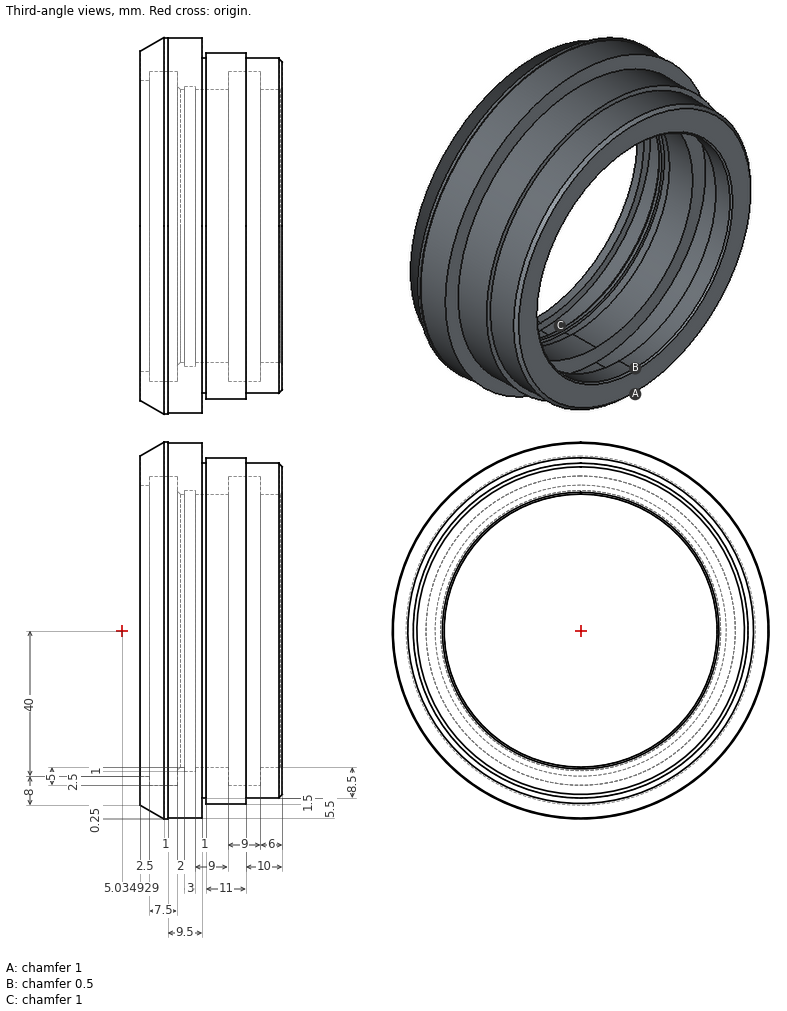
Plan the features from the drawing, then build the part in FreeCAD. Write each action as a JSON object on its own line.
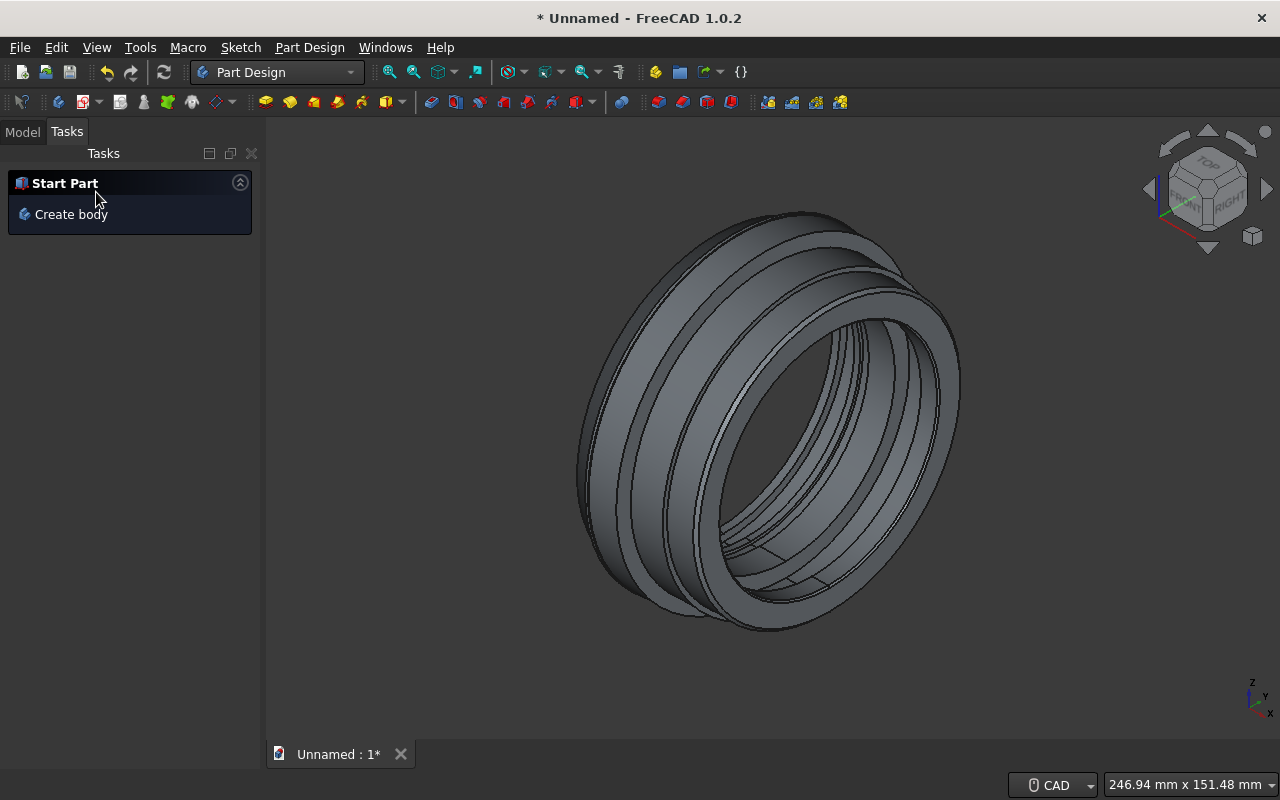
{"action": "key", "text": "2"}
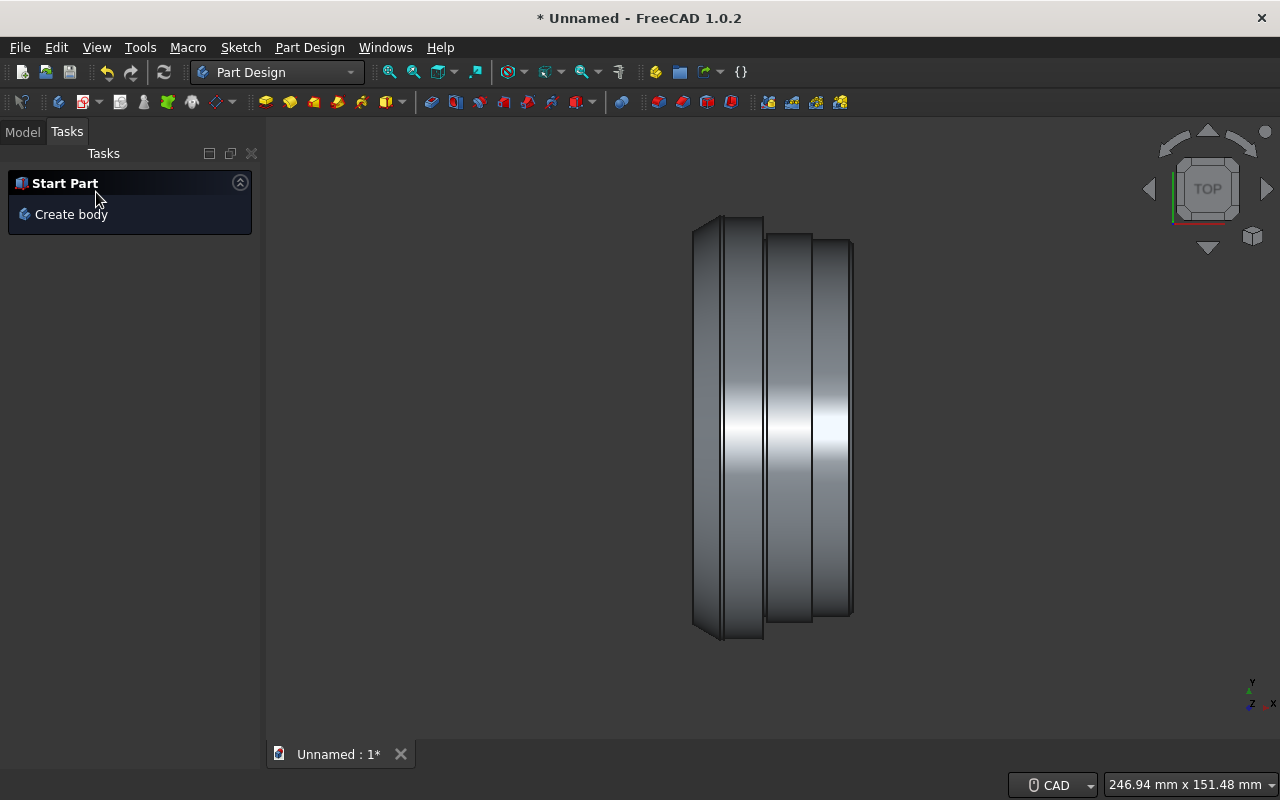
{"action": "key", "text": "1"}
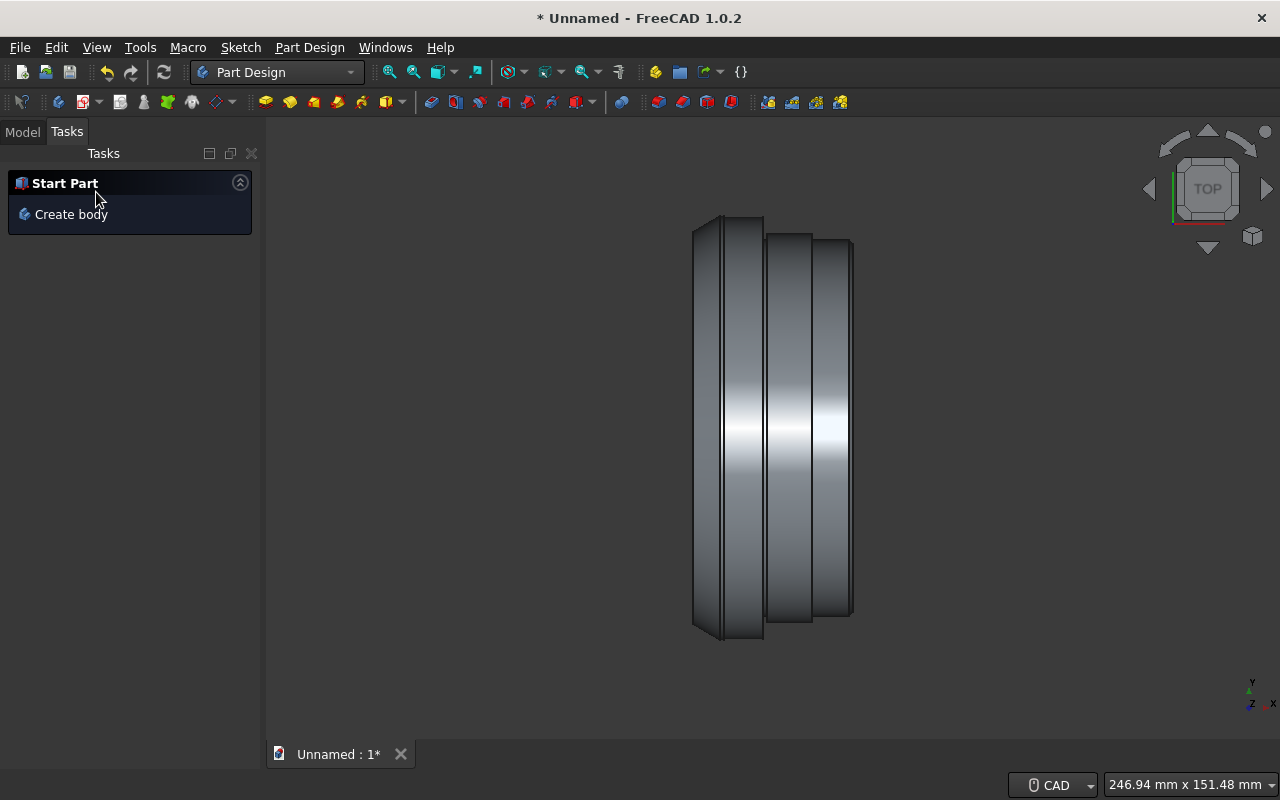
{"action": "key", "text": "3"}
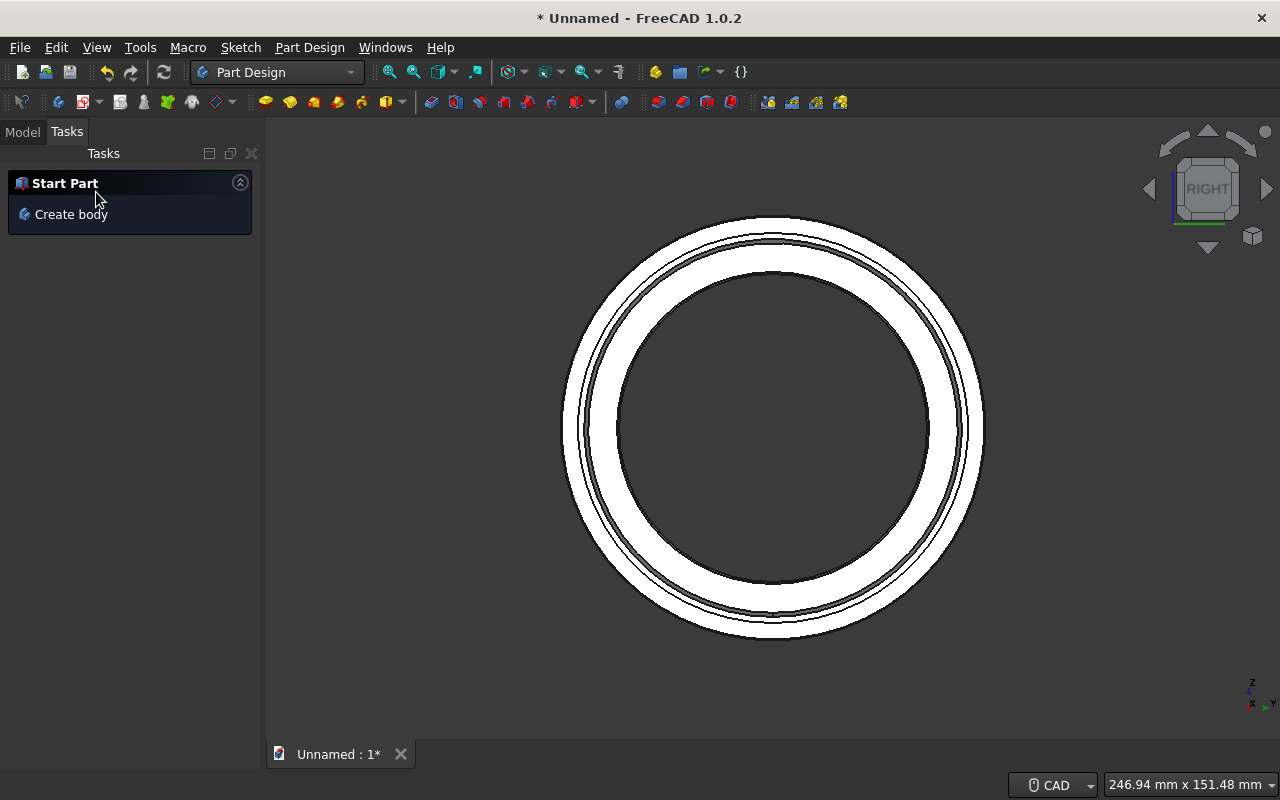
{"action": "key", "text": "5"}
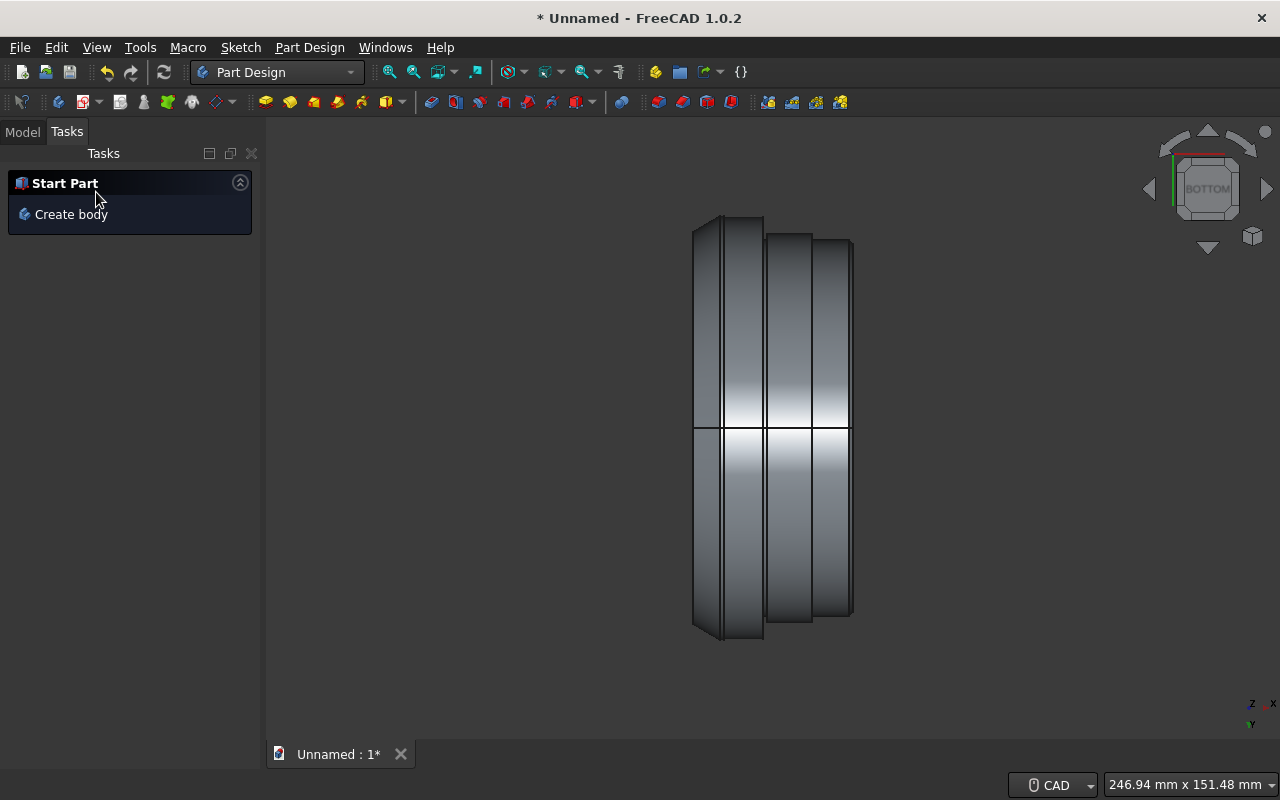
{"action": "key", "text": "4"}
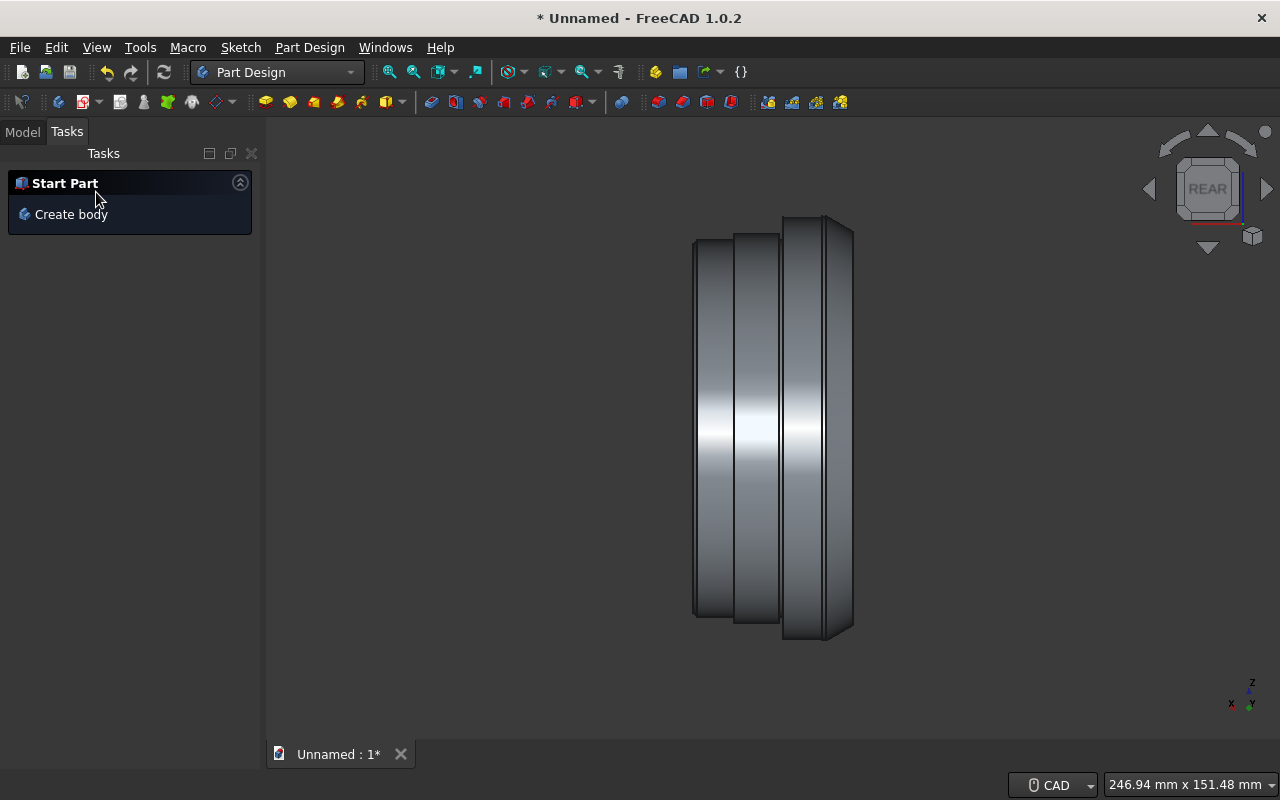
{"action": "key", "text": "6"}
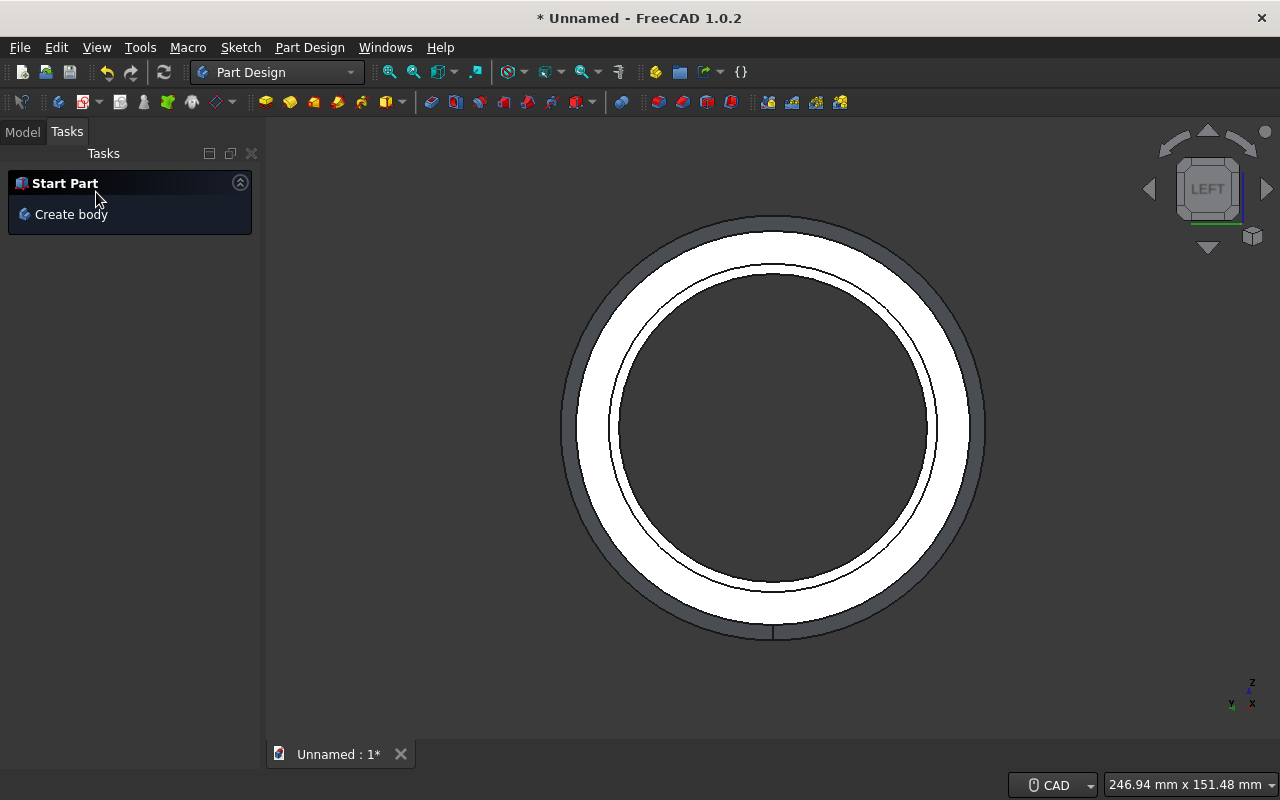
{"action": "left_click", "coordinate": [773, 273]}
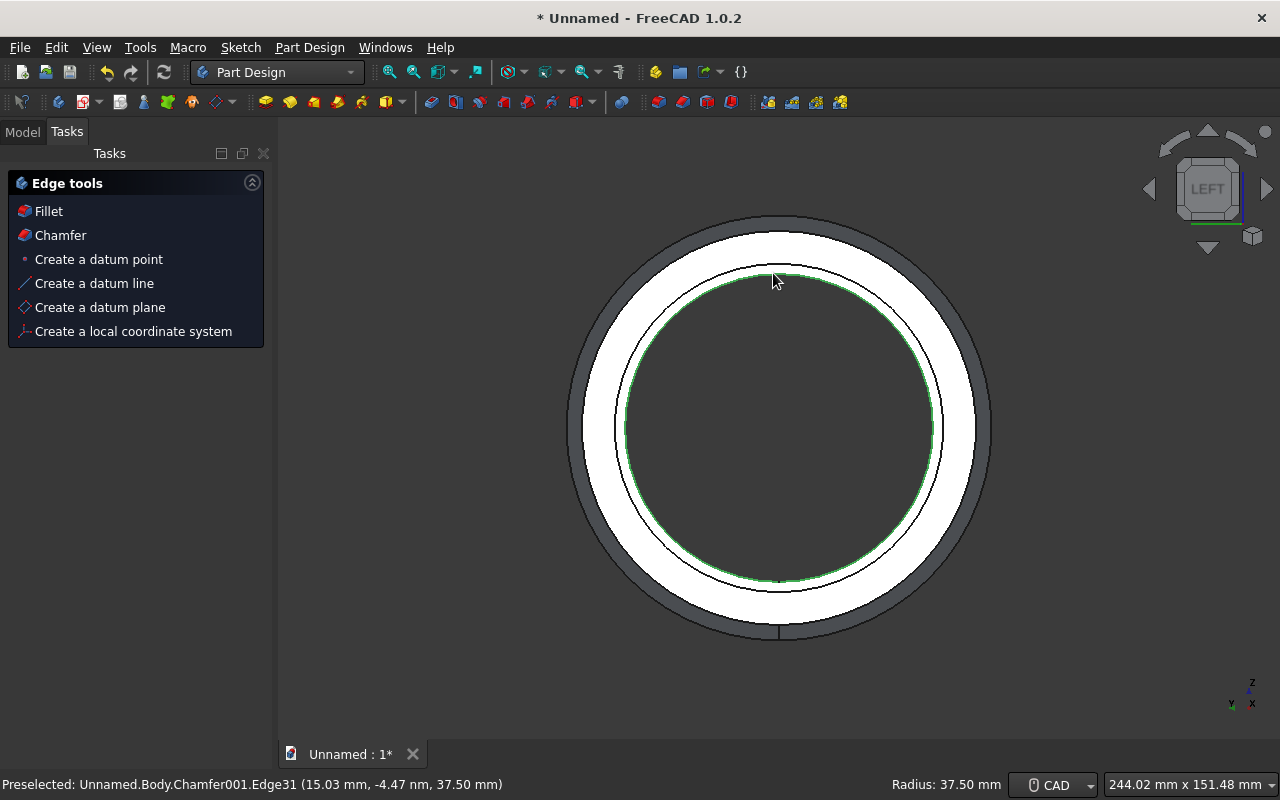
{"action": "left_click", "coordinate": [684, 102]}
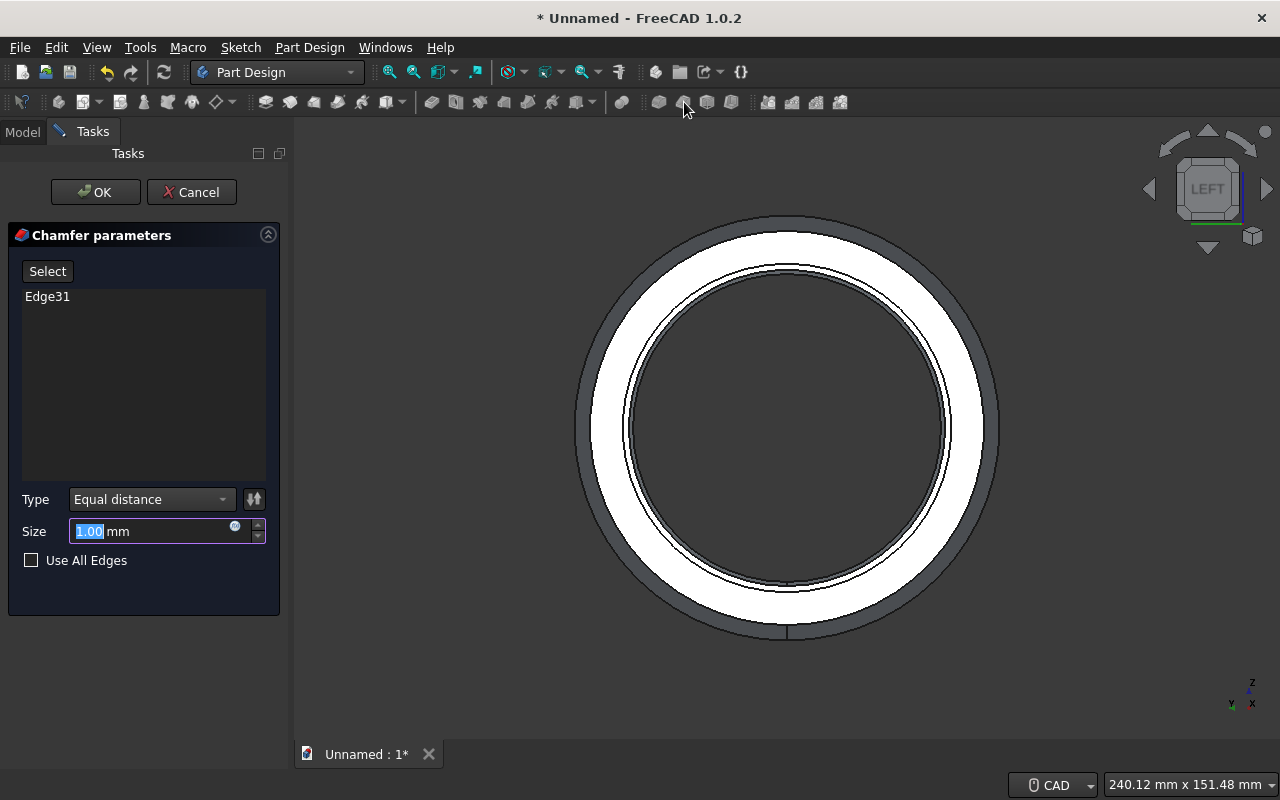
{"action": "type", "text": "1"}
{"action": "key", "text": "Tab"}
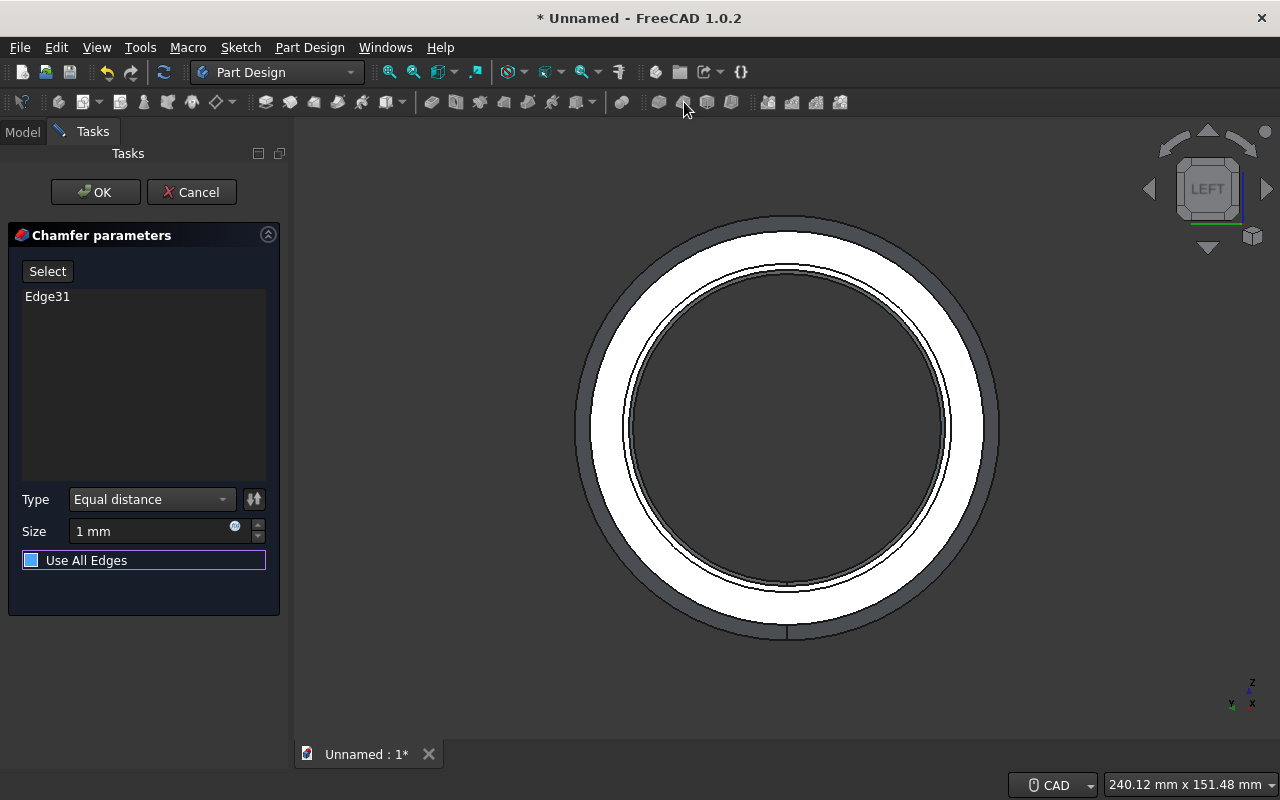
{"action": "left_click", "coordinate": [96, 192]}